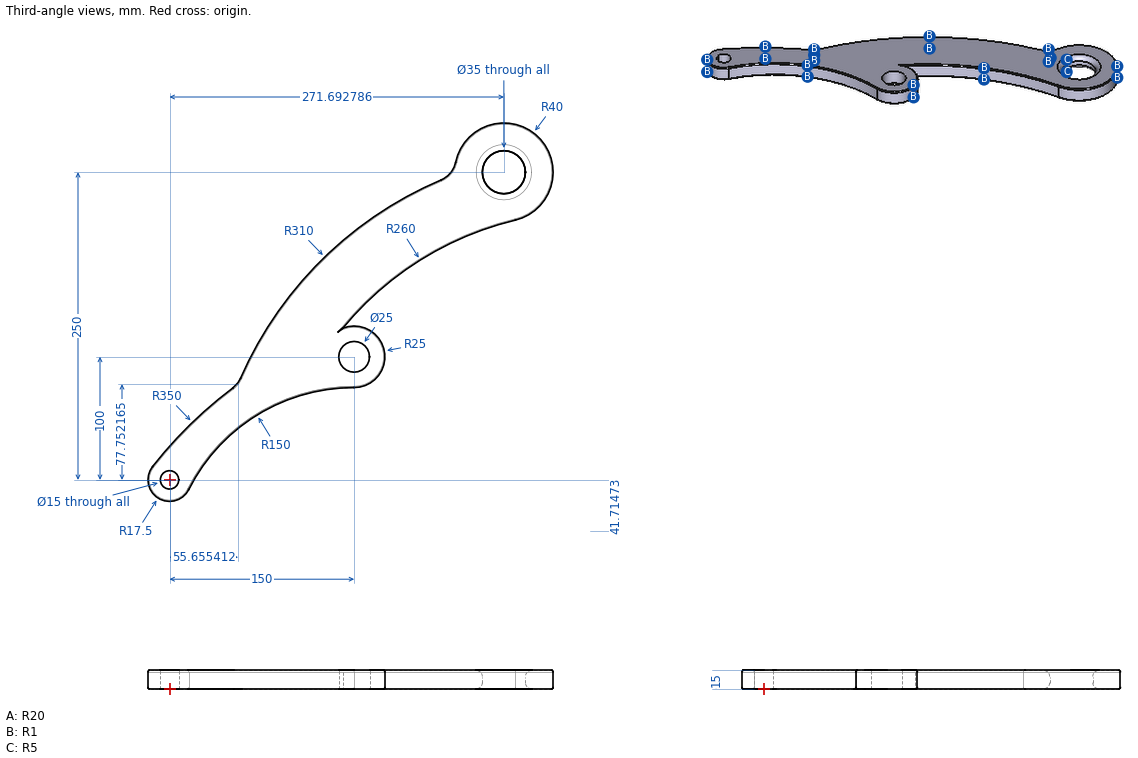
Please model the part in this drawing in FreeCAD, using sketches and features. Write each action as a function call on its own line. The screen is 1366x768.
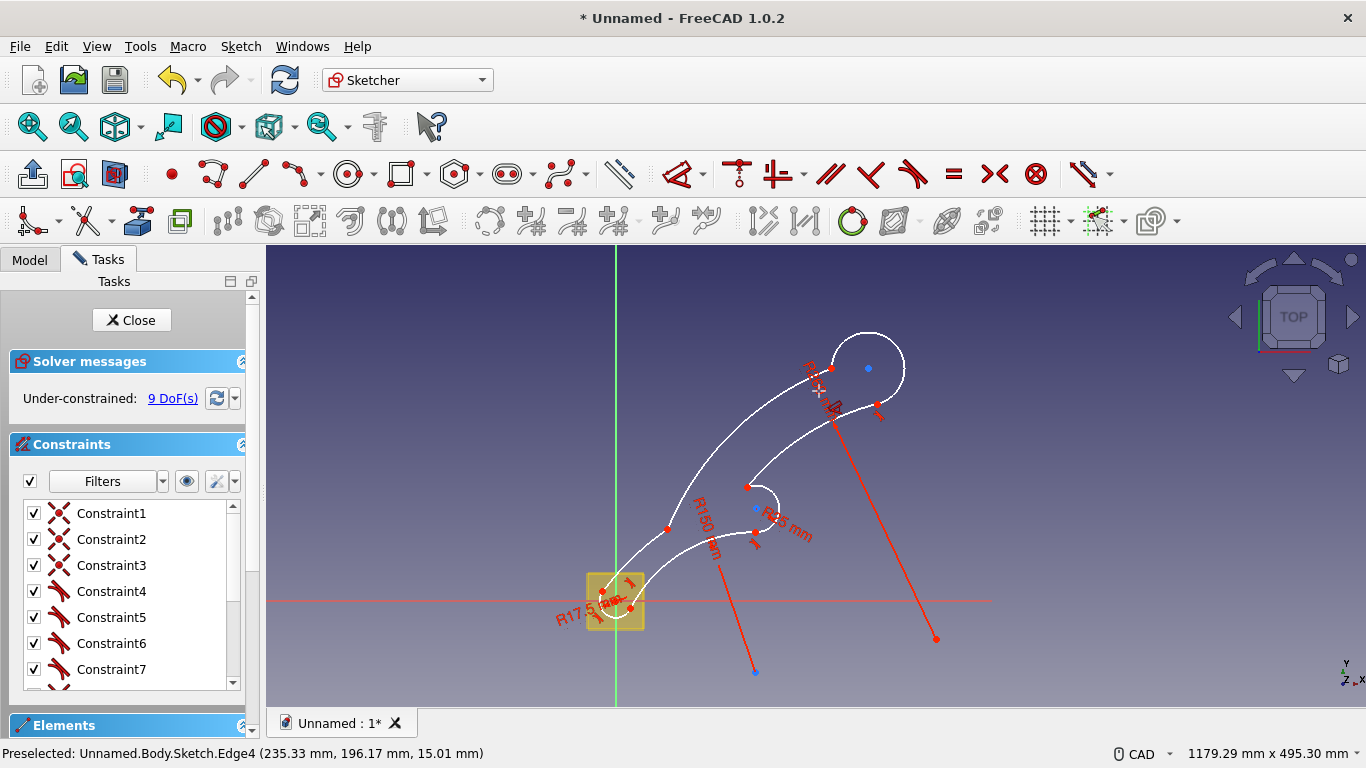
click(904, 368)
click(936, 367)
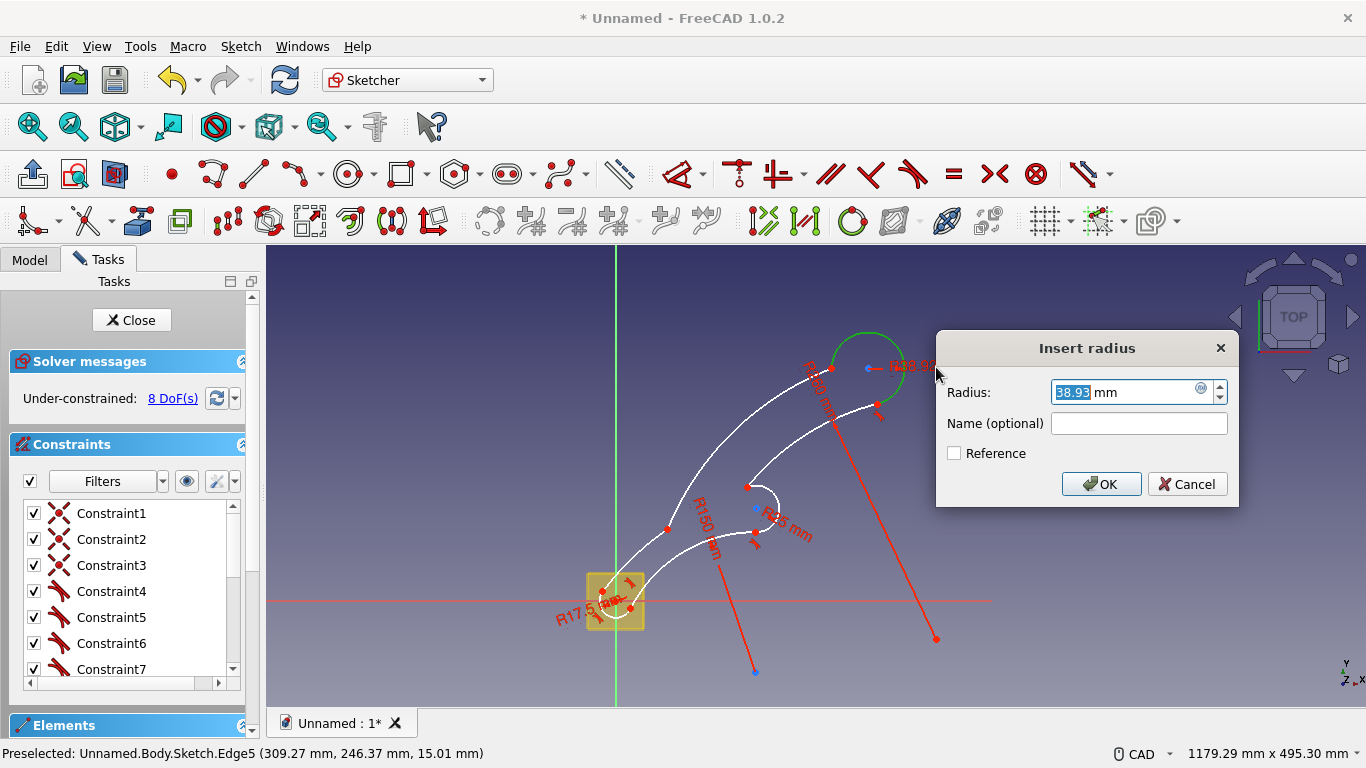
text(40)
key(Return)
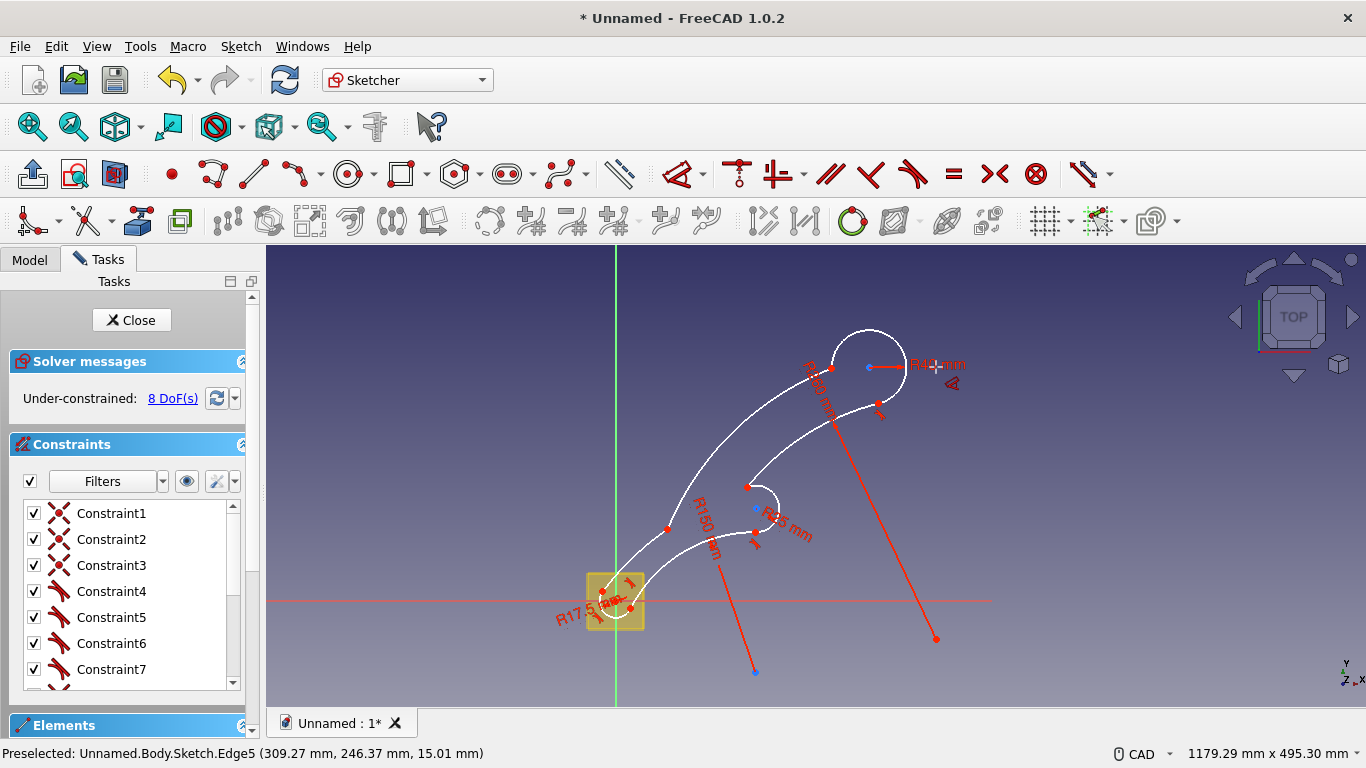
click(769, 402)
click(900, 319)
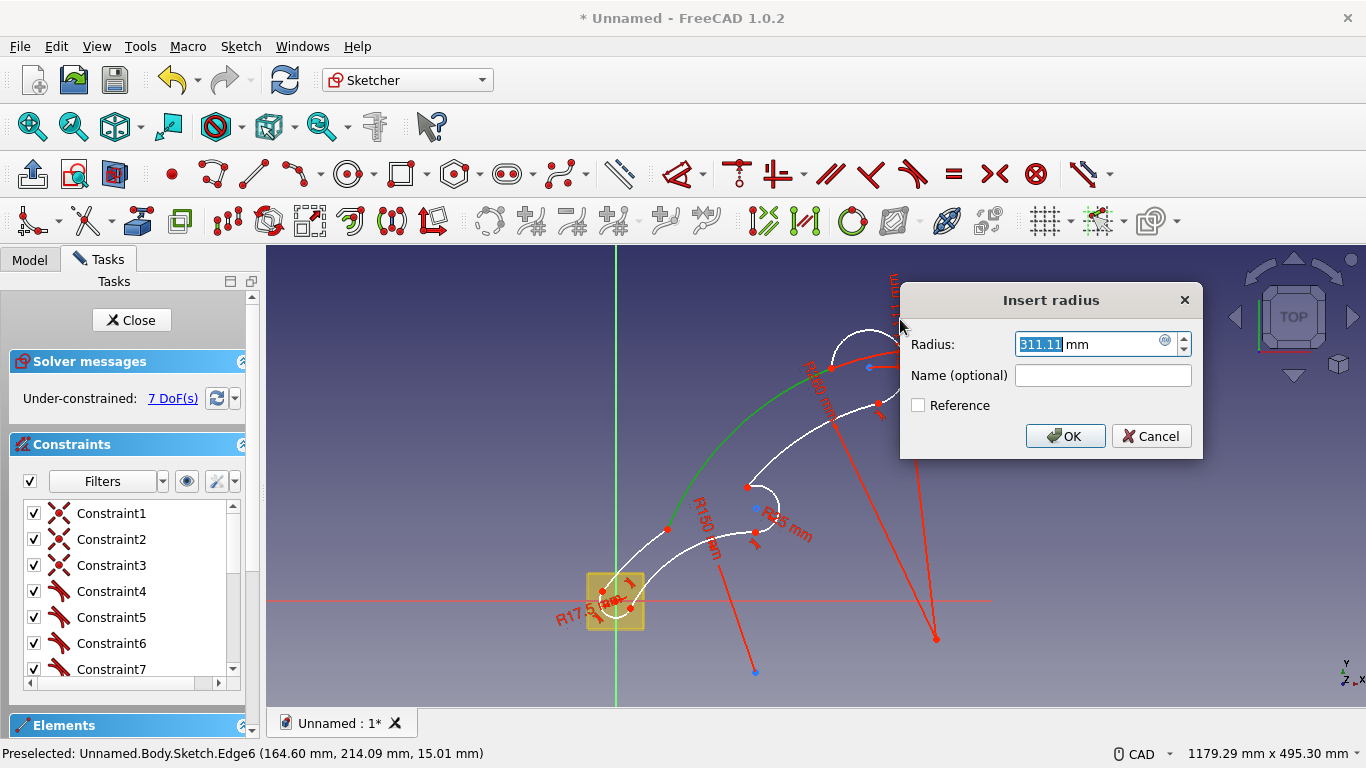
text(310)
key(Return)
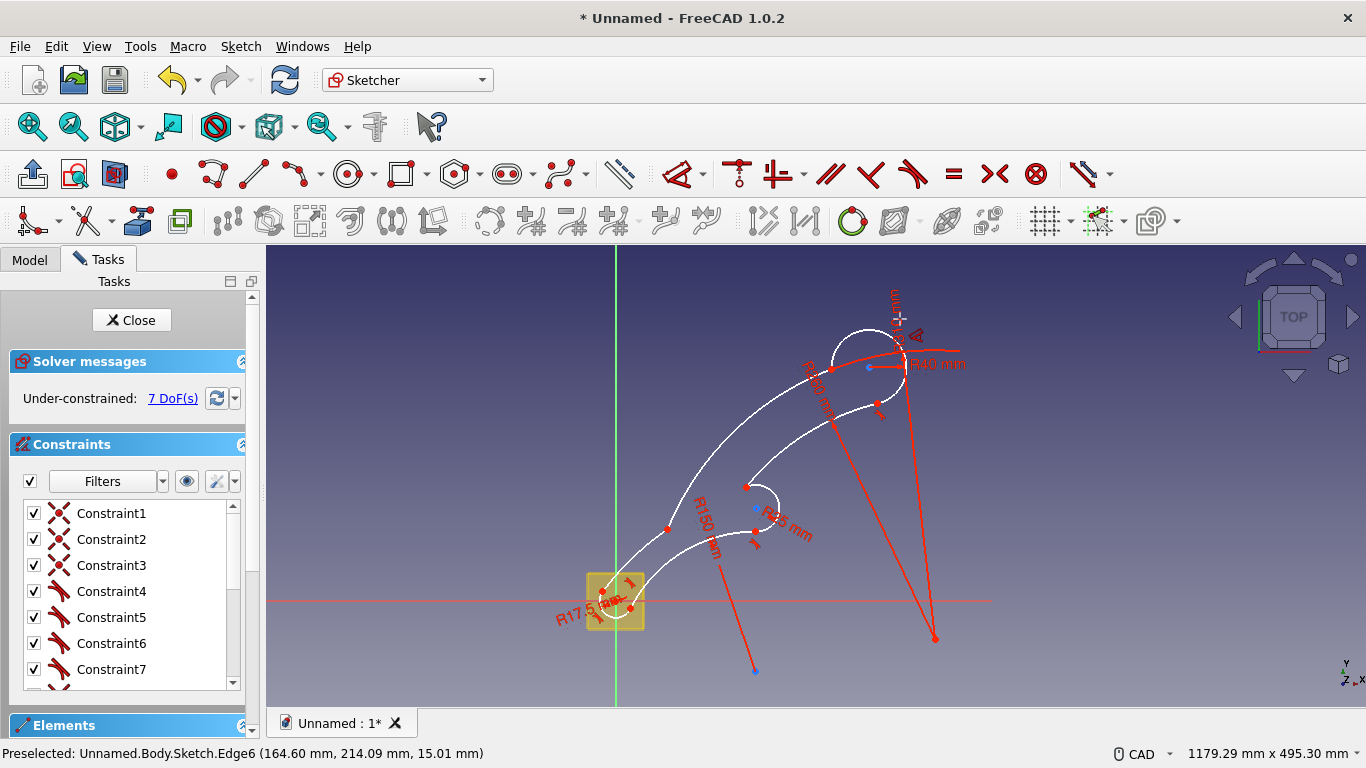
click(646, 546)
click(537, 645)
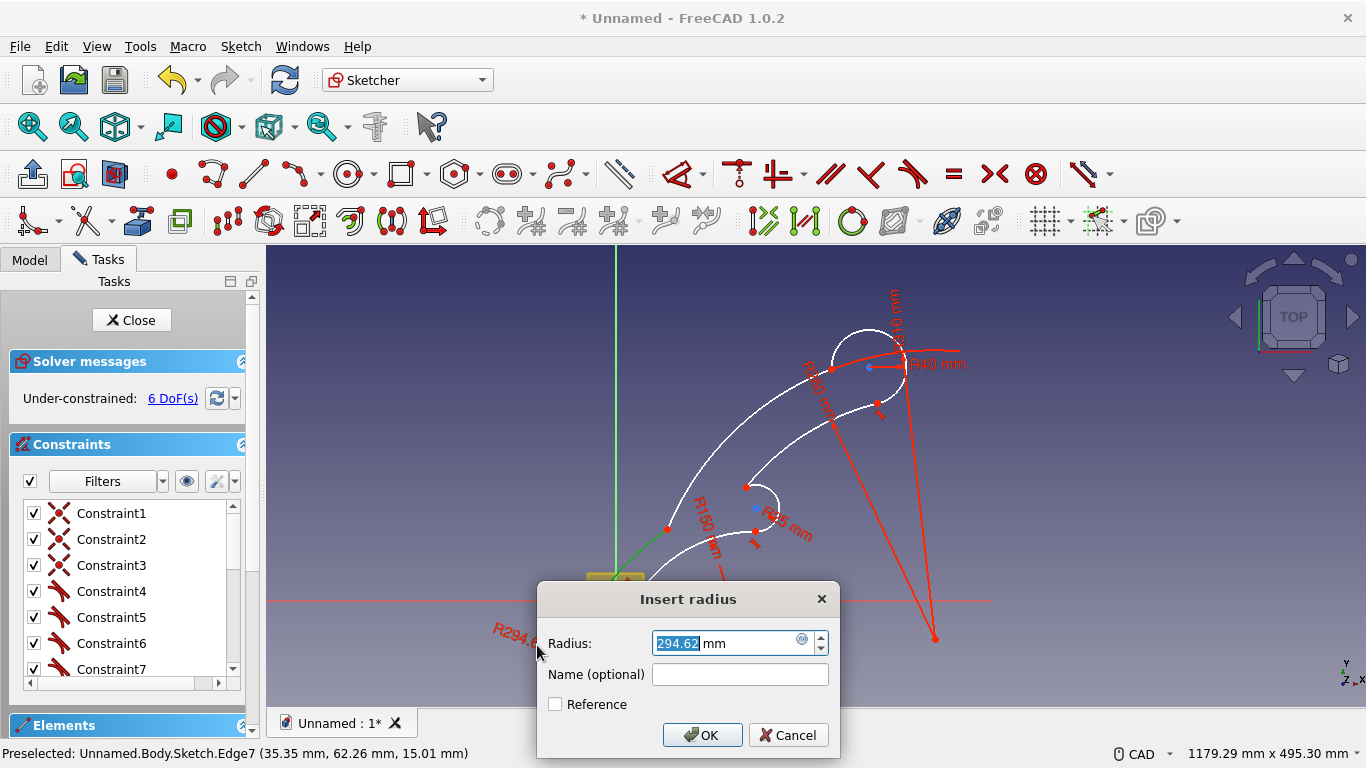
text(350)
key(Return)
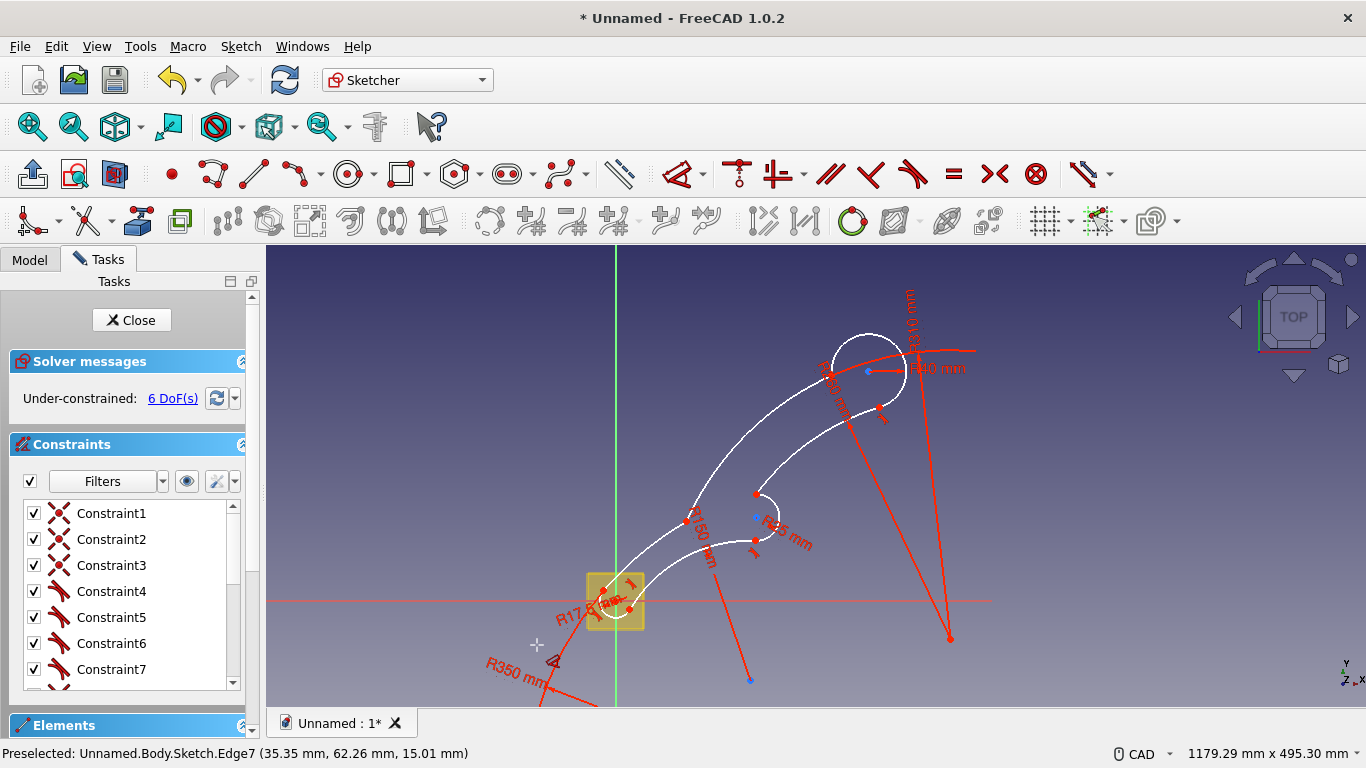
click(756, 517)
click(686, 635)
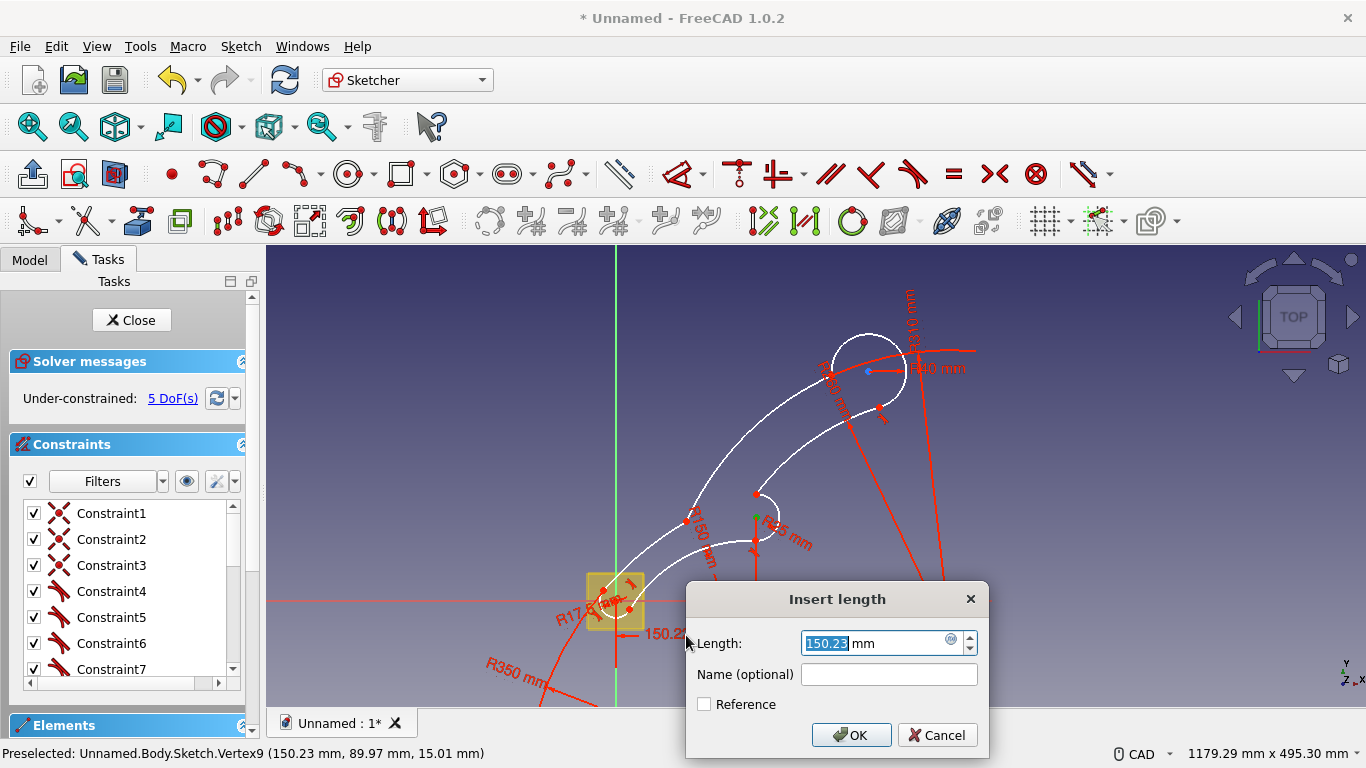
text(150)
key(Return)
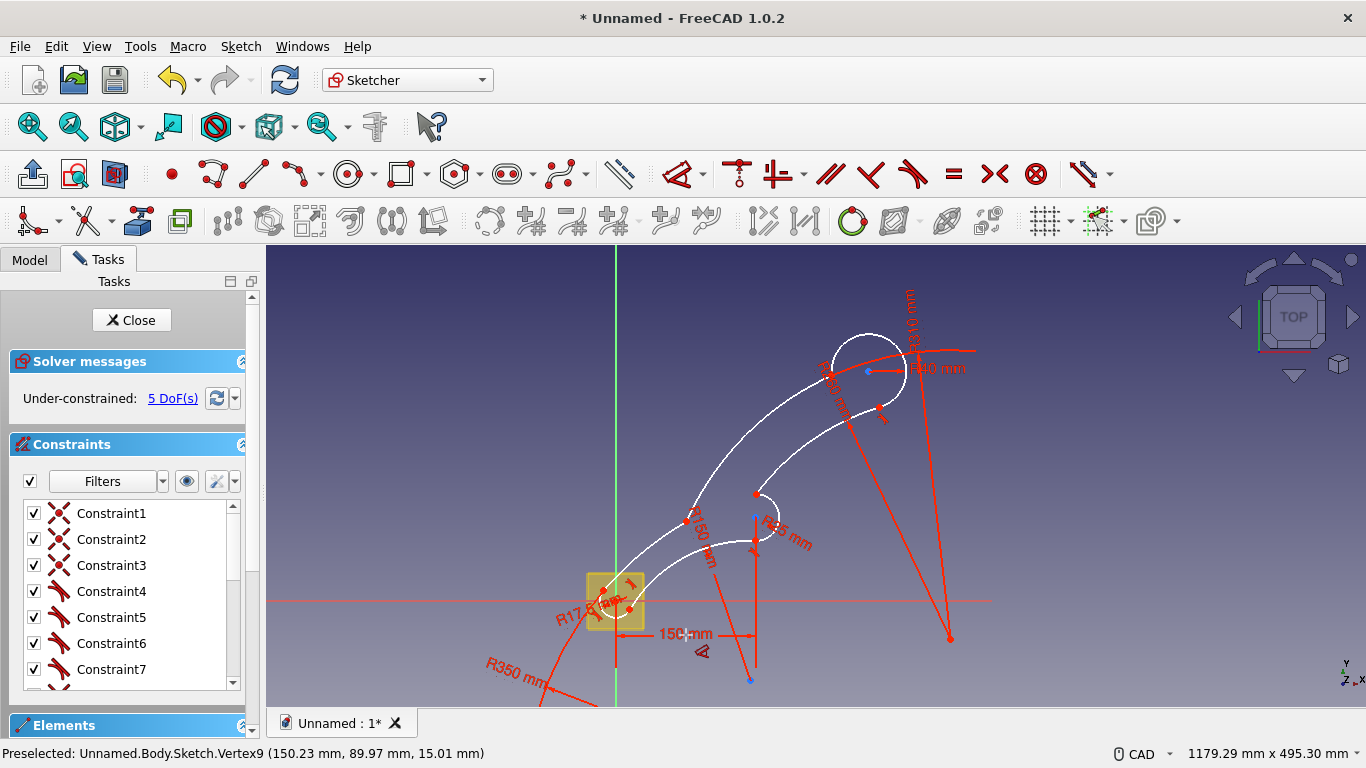
click(756, 517)
click(582, 559)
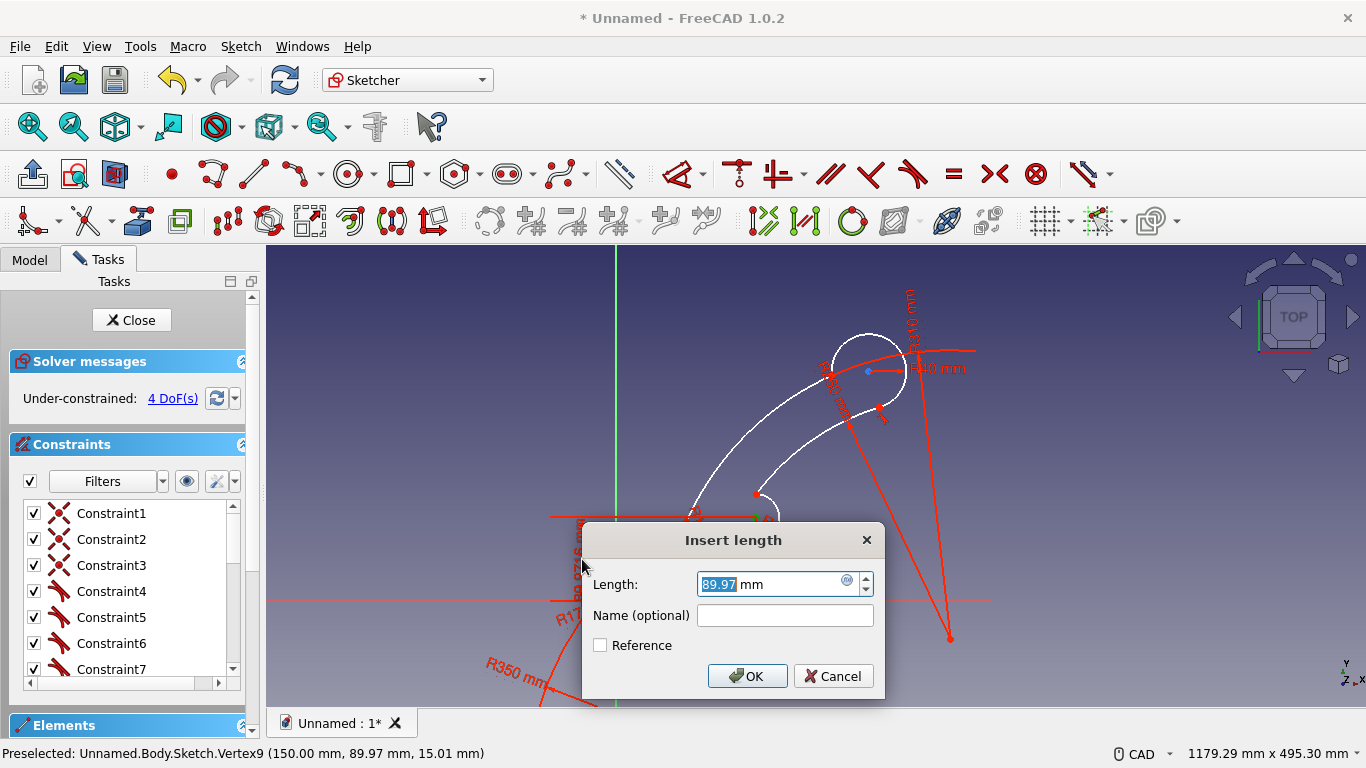
text(100)
key(Return)